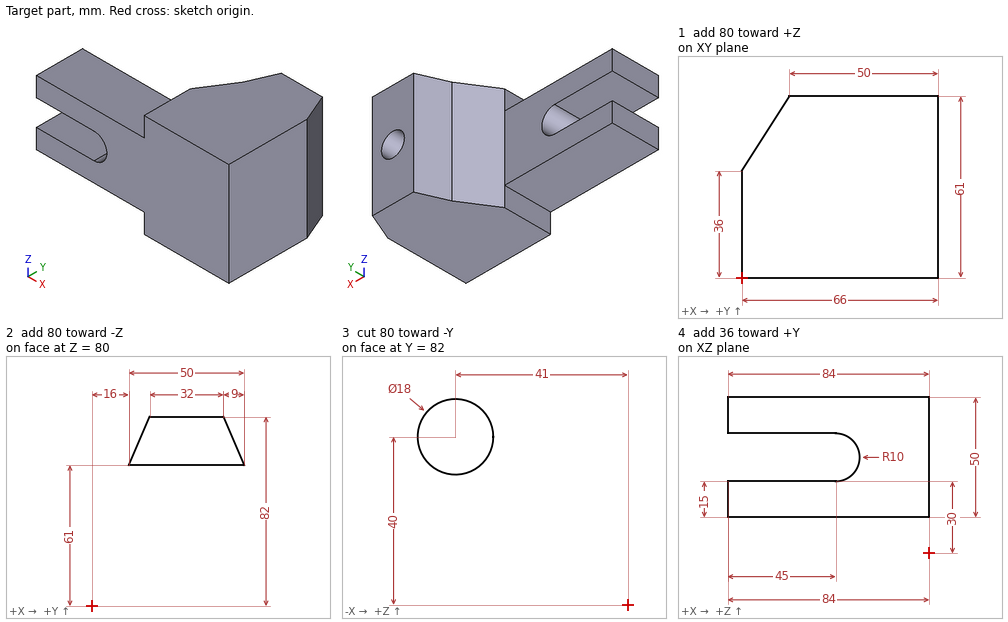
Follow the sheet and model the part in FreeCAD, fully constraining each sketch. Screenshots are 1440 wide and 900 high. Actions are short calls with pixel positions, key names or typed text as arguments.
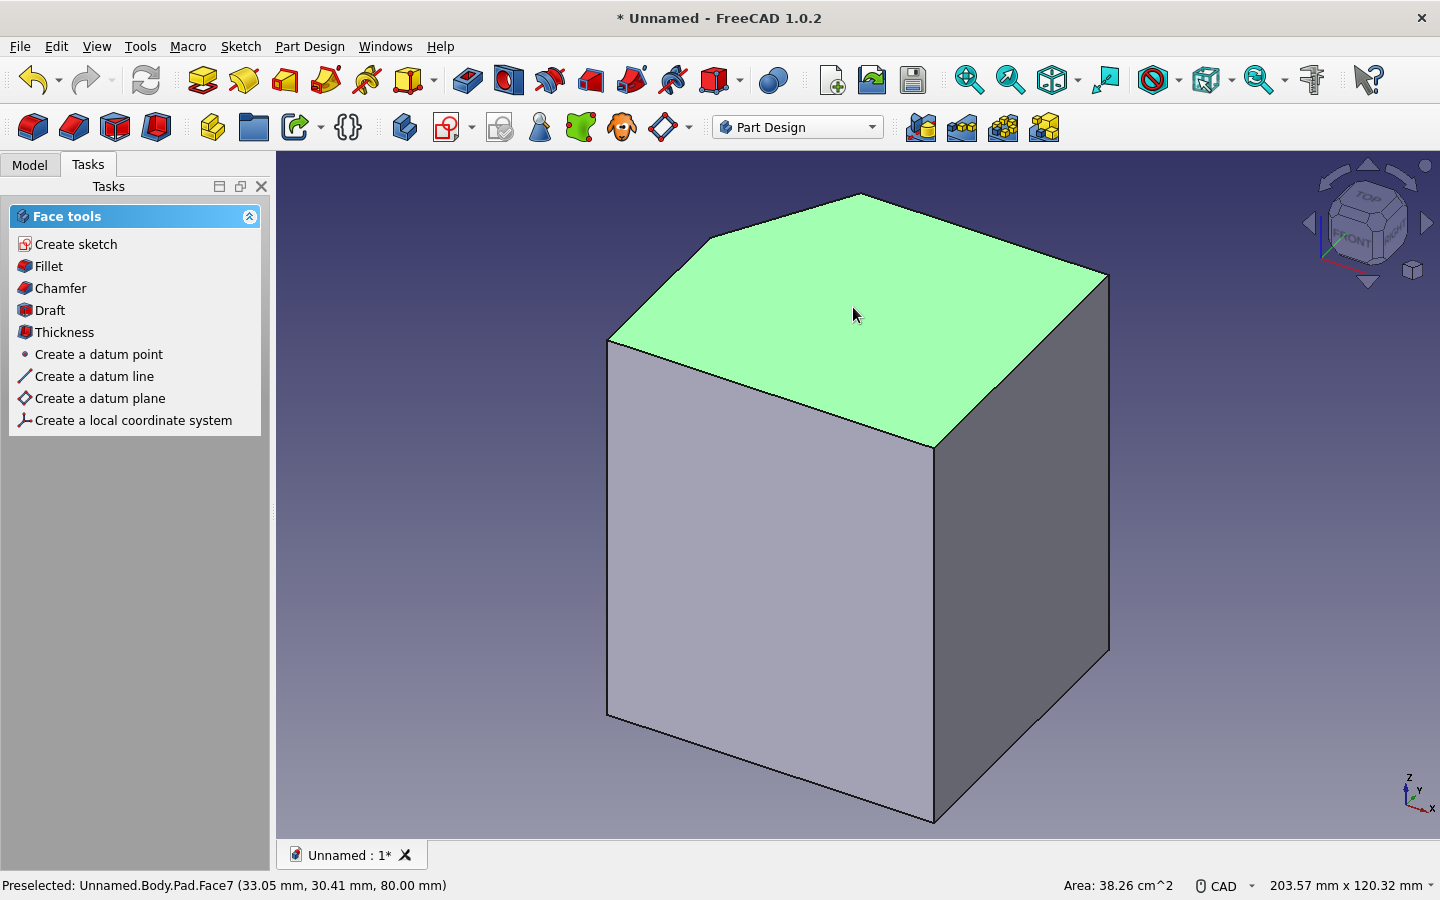
click(446, 128)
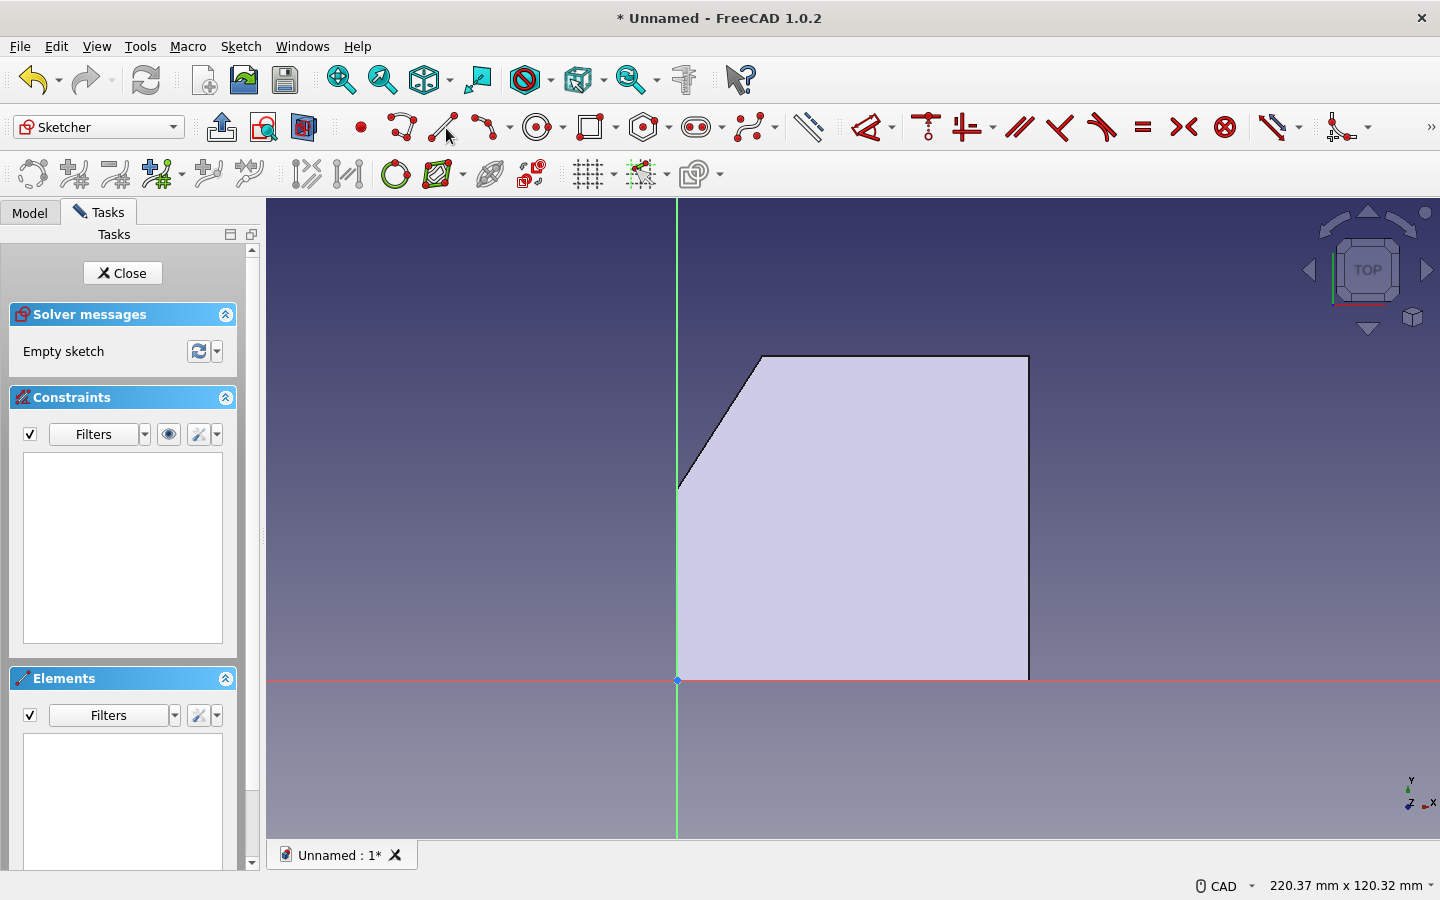
scroll(475, 771, down, 1)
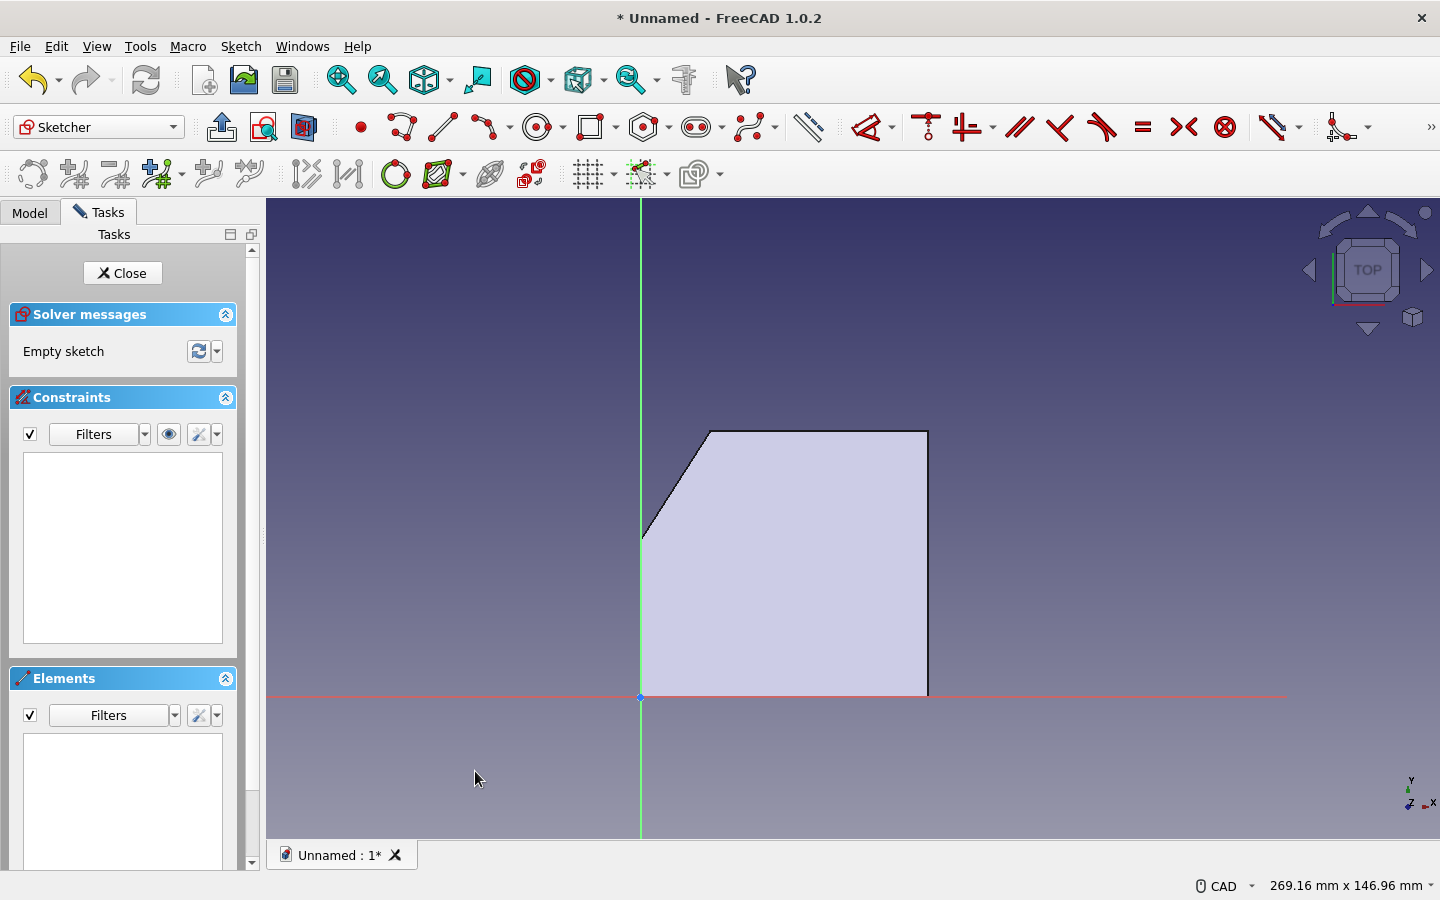
key(g)
key(m)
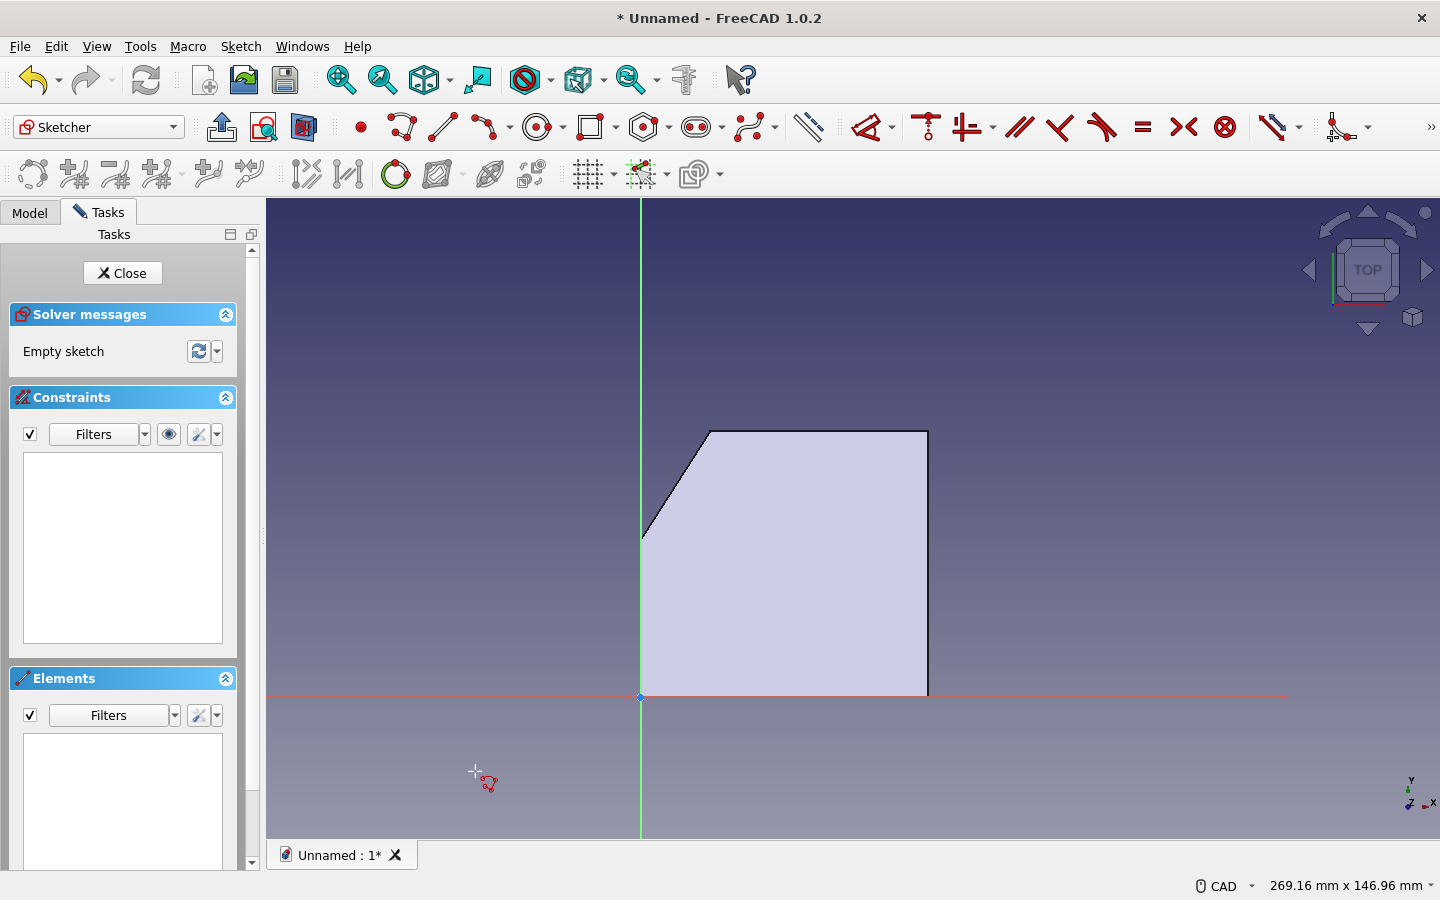
click(710, 431)
click(928, 431)
click(889, 340)
click(750, 340)
click(710, 432)
key(Escape)
key(Escape)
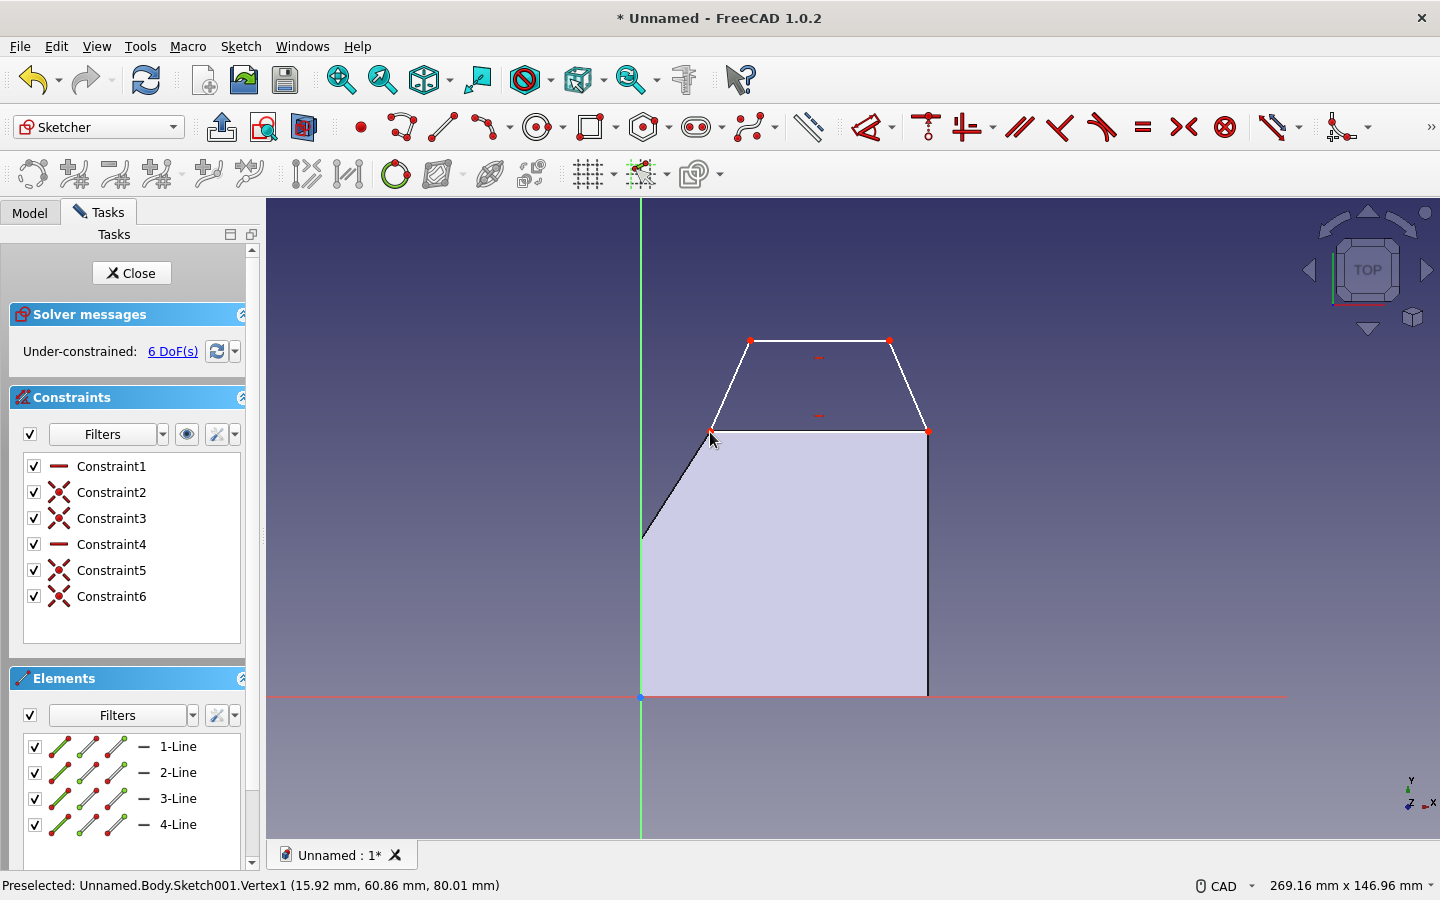
click(866, 128)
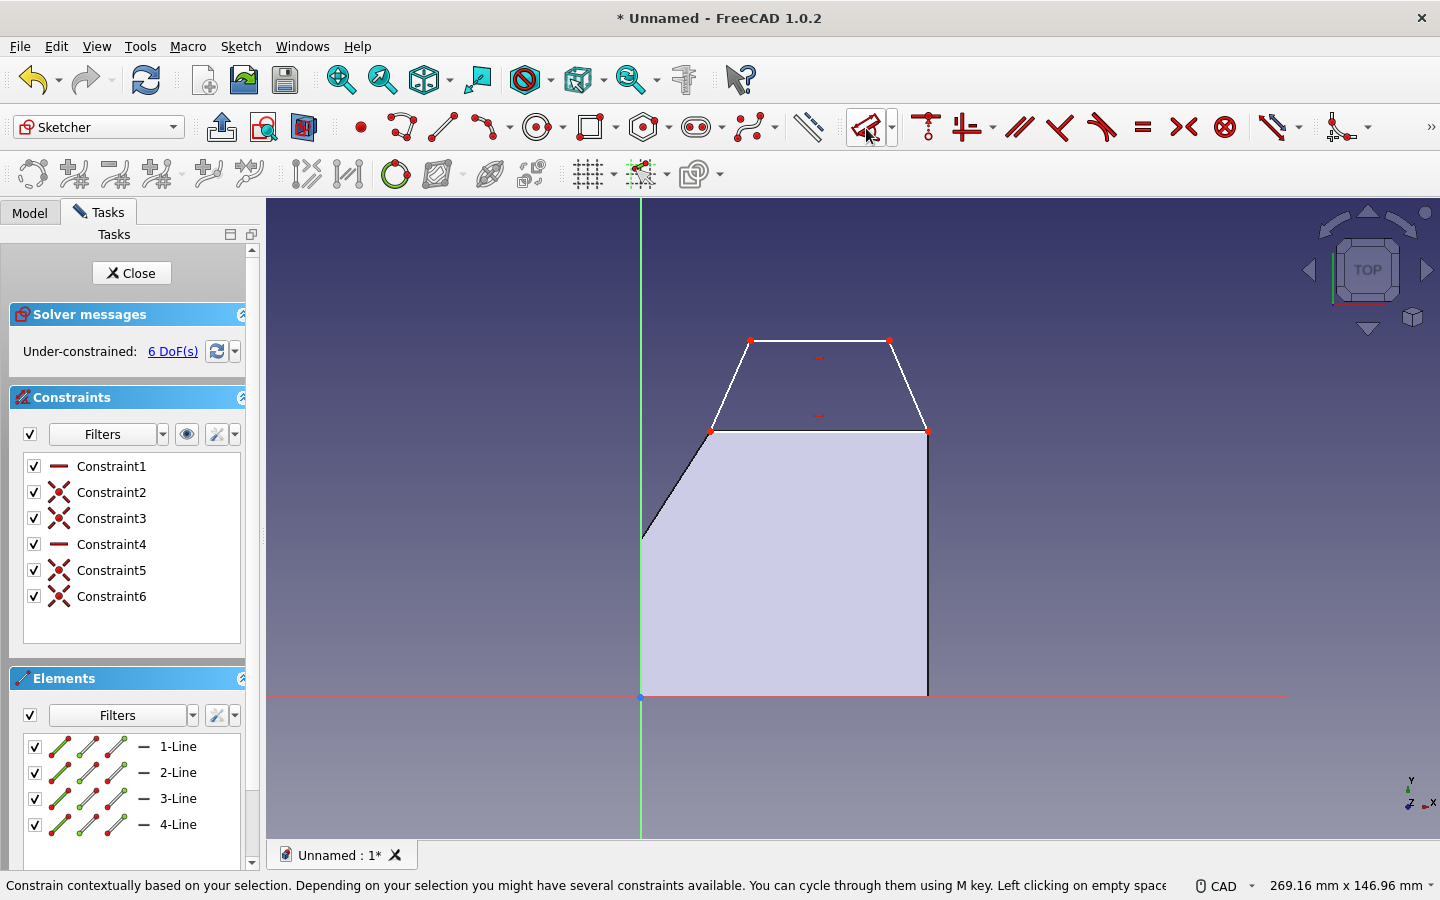
click(775, 432)
click(819, 398)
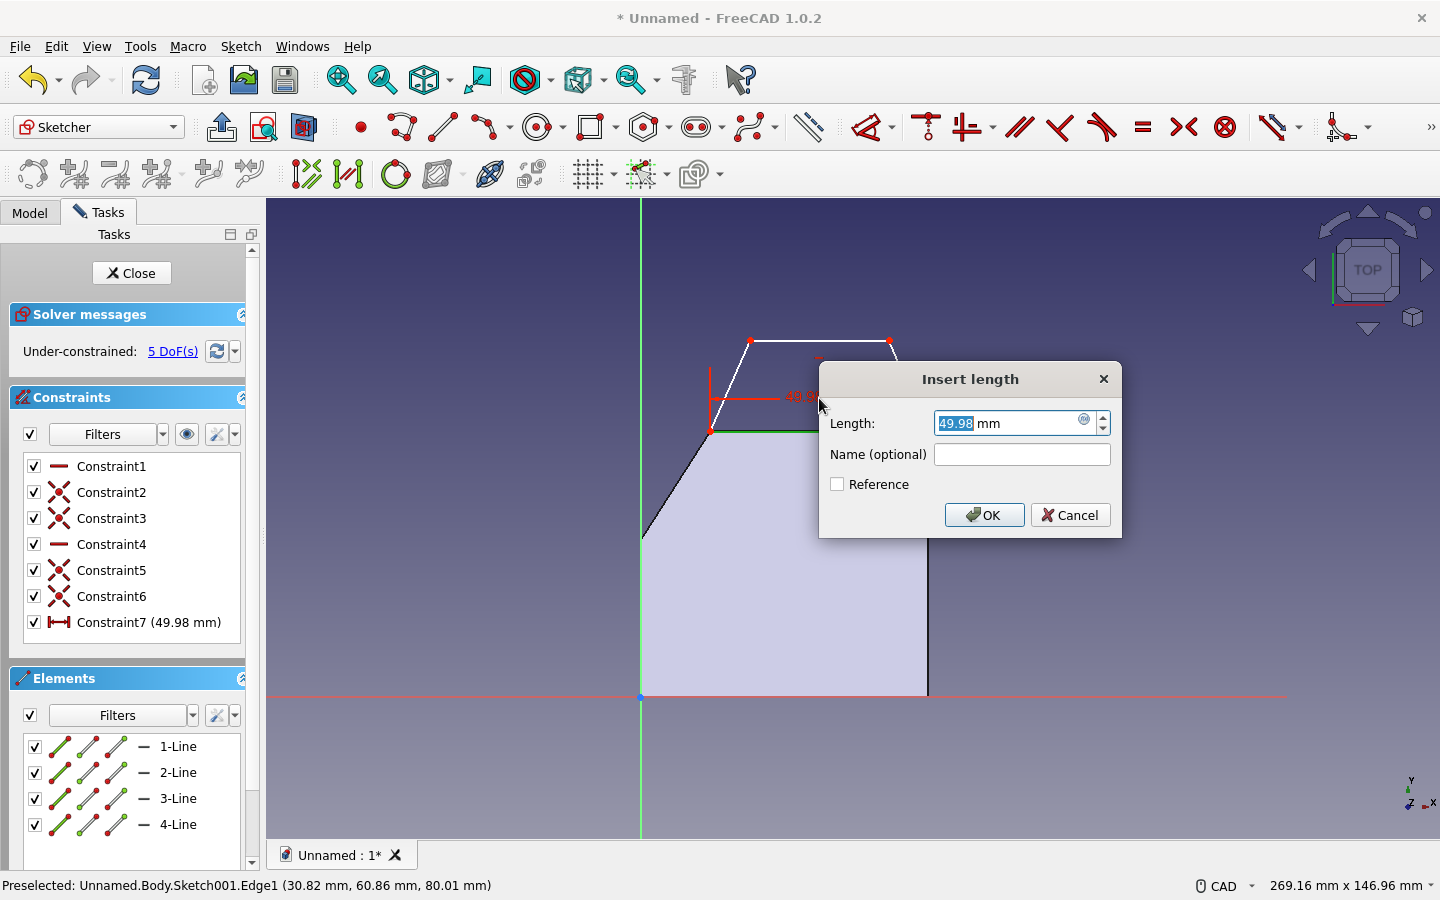
text(50)
key(Return)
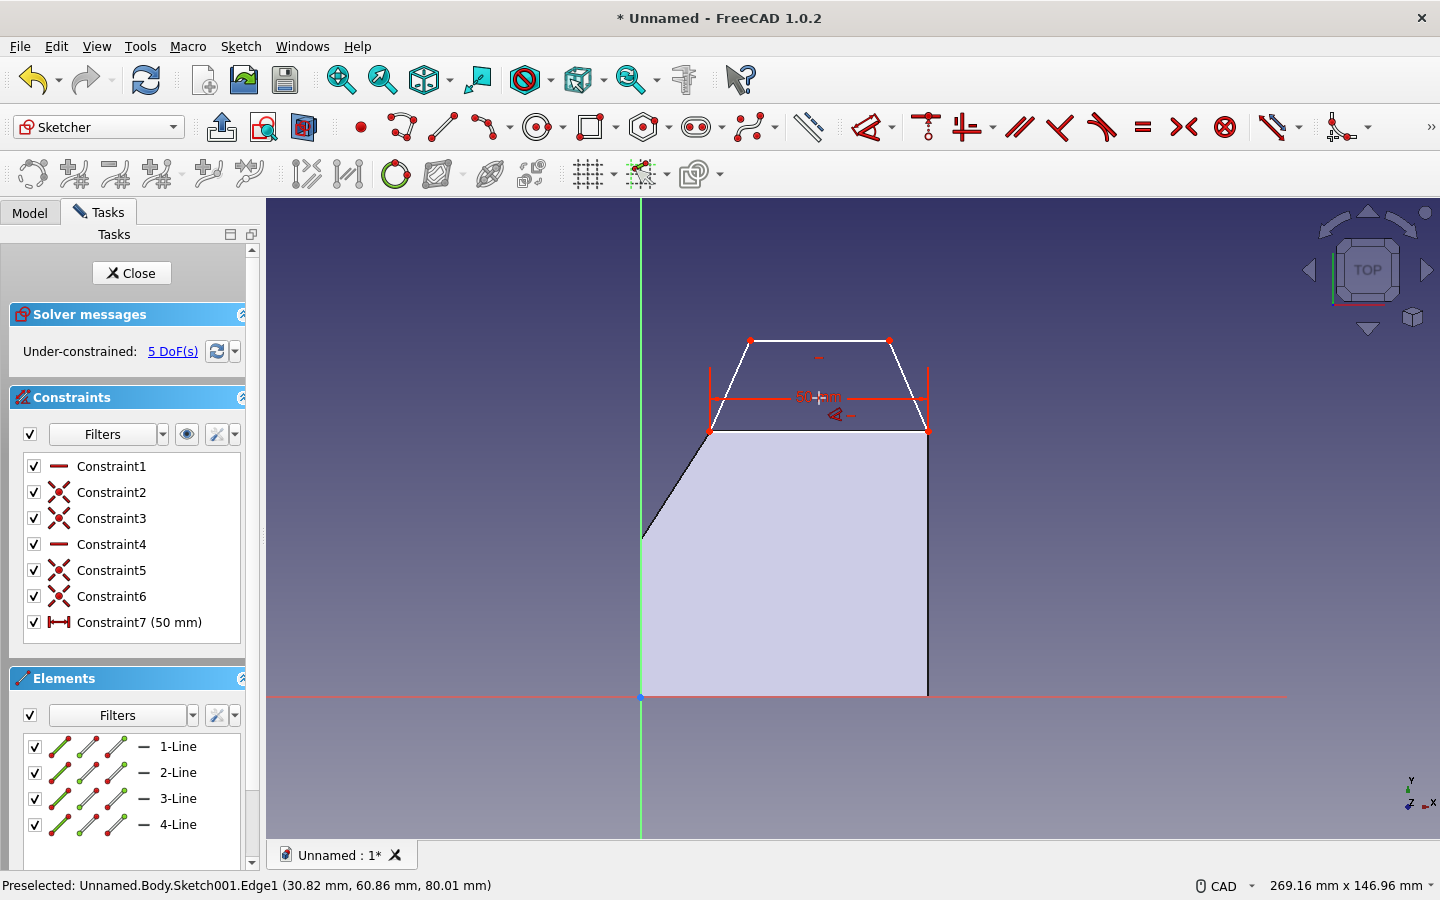
click(847, 341)
click(819, 307)